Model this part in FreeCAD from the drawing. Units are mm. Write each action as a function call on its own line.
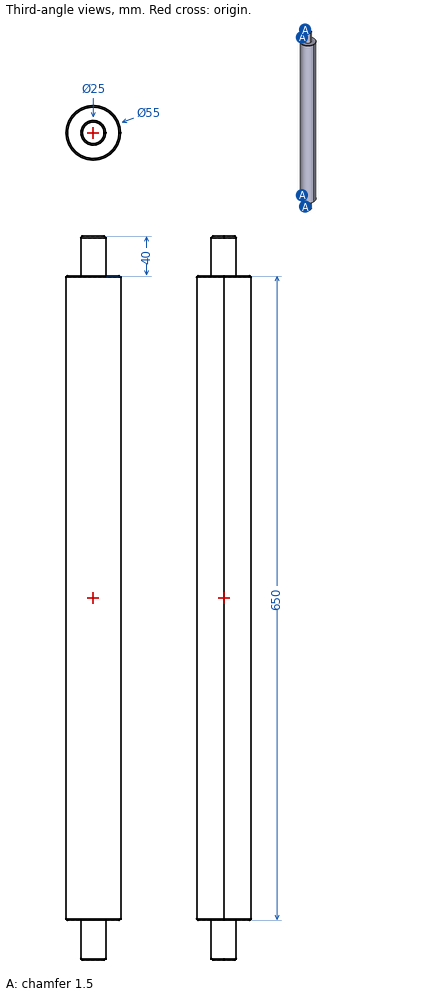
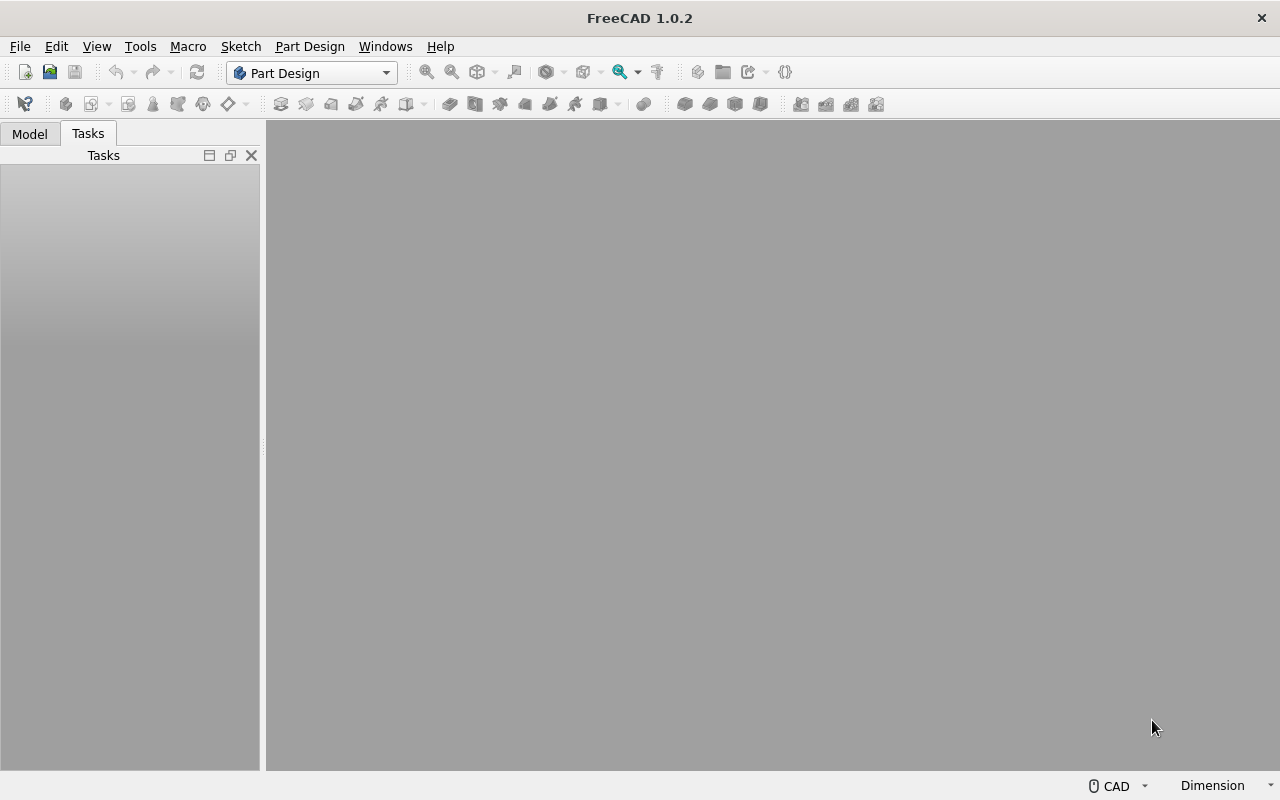
click(25, 72)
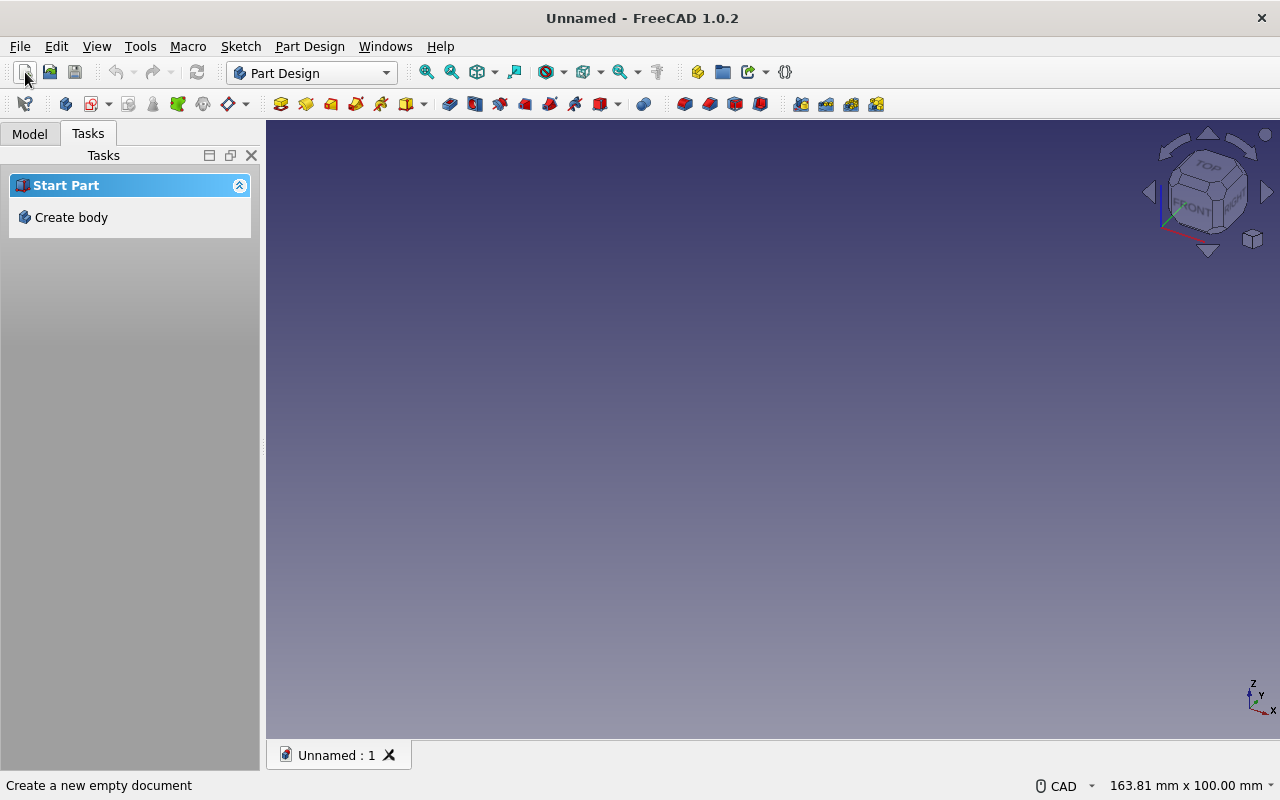
click(90, 104)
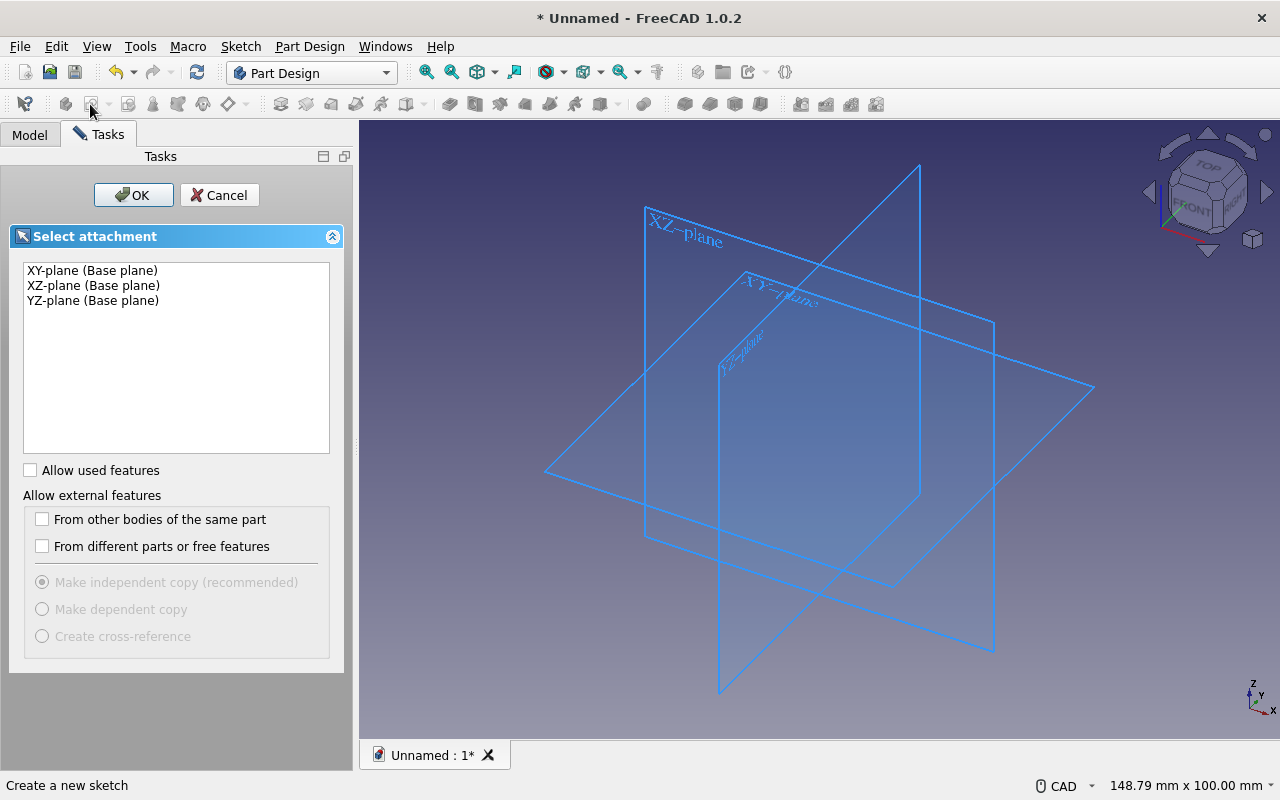
click(84, 270)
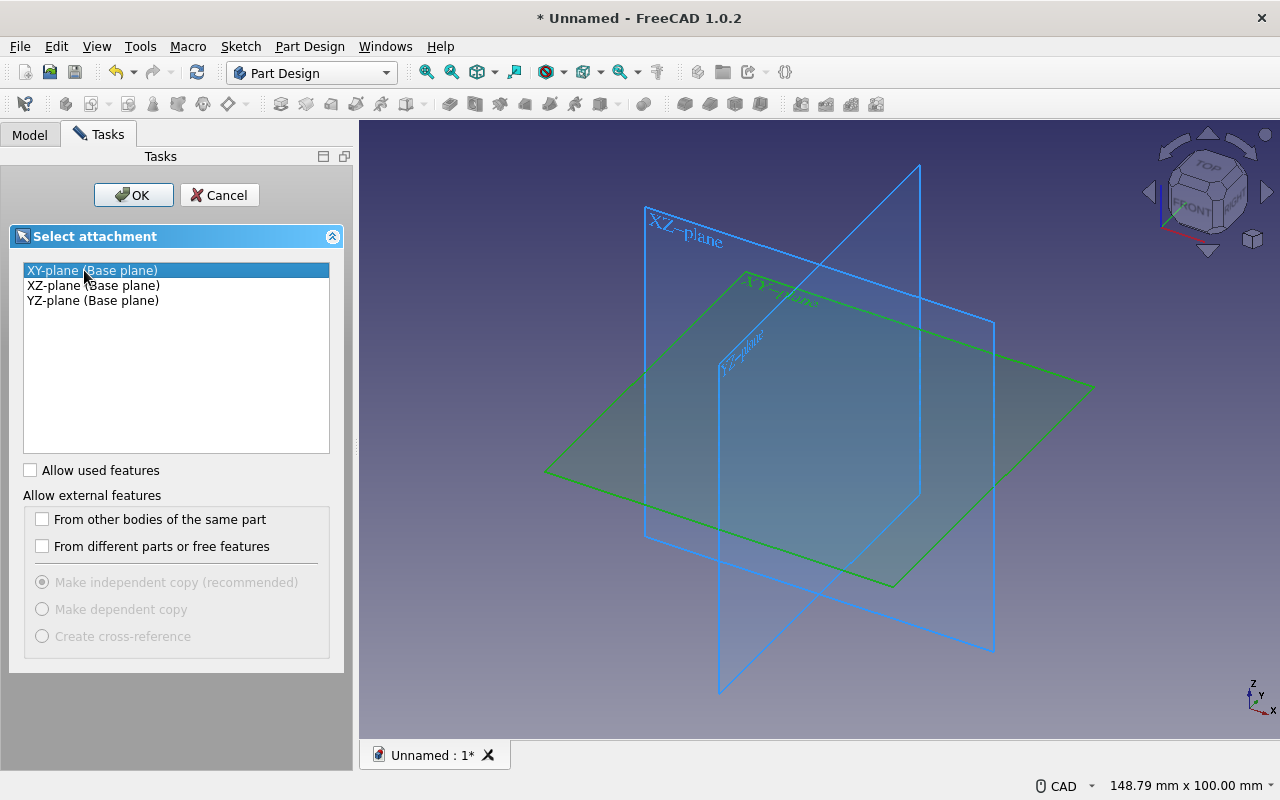
click(134, 195)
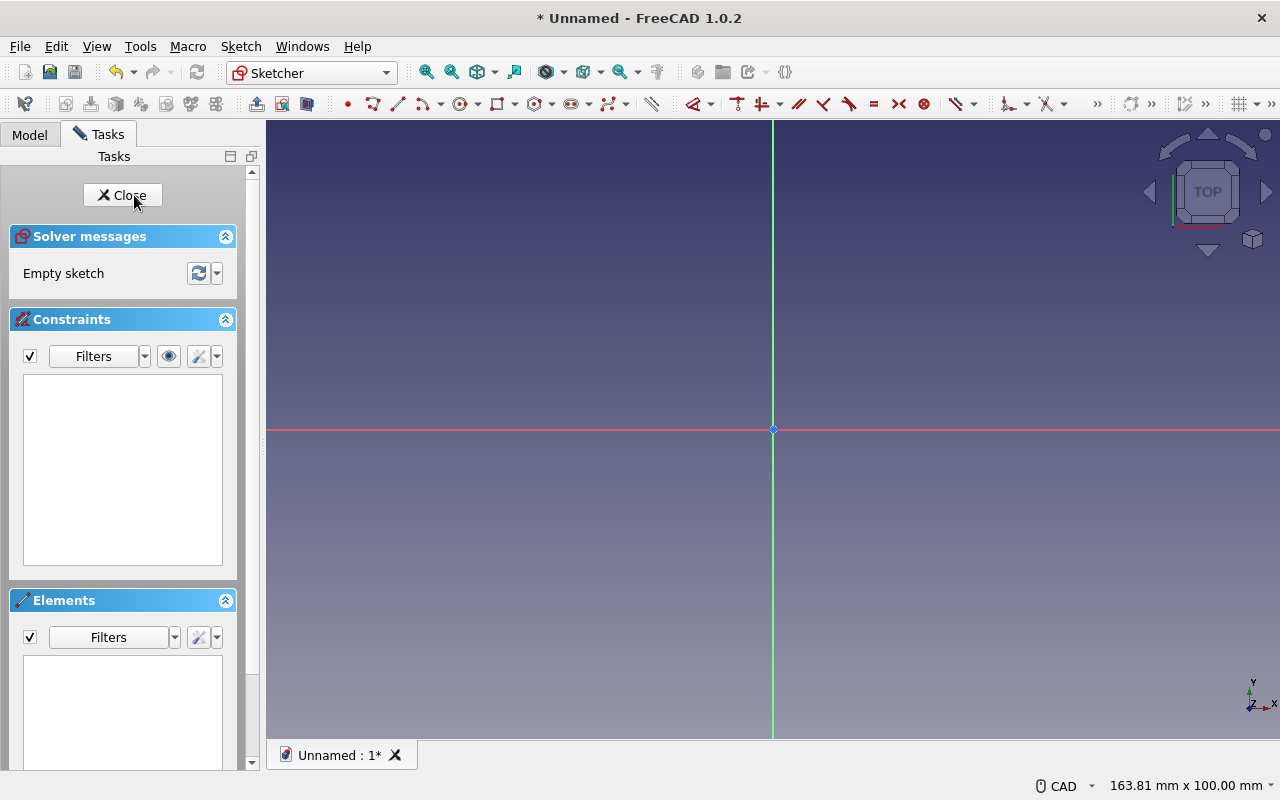
click(460, 104)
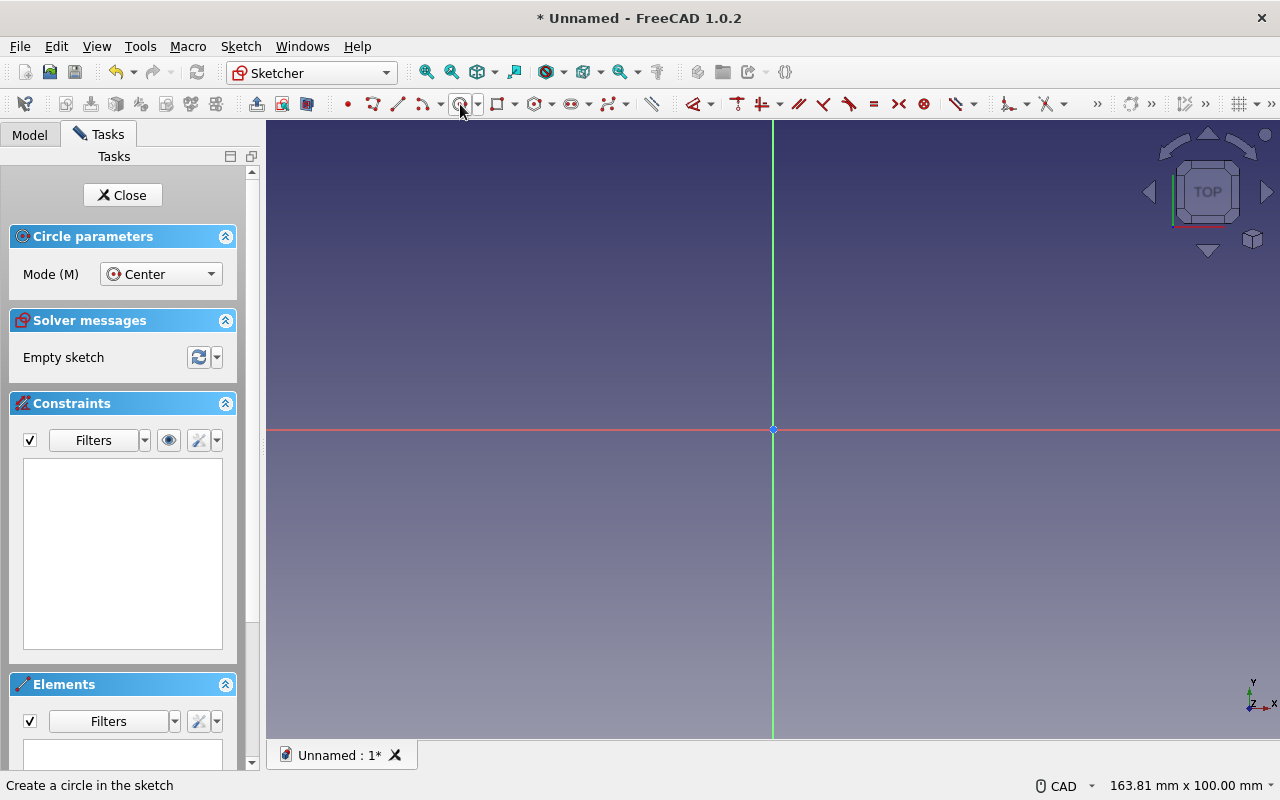
click(773, 430)
move(893, 309)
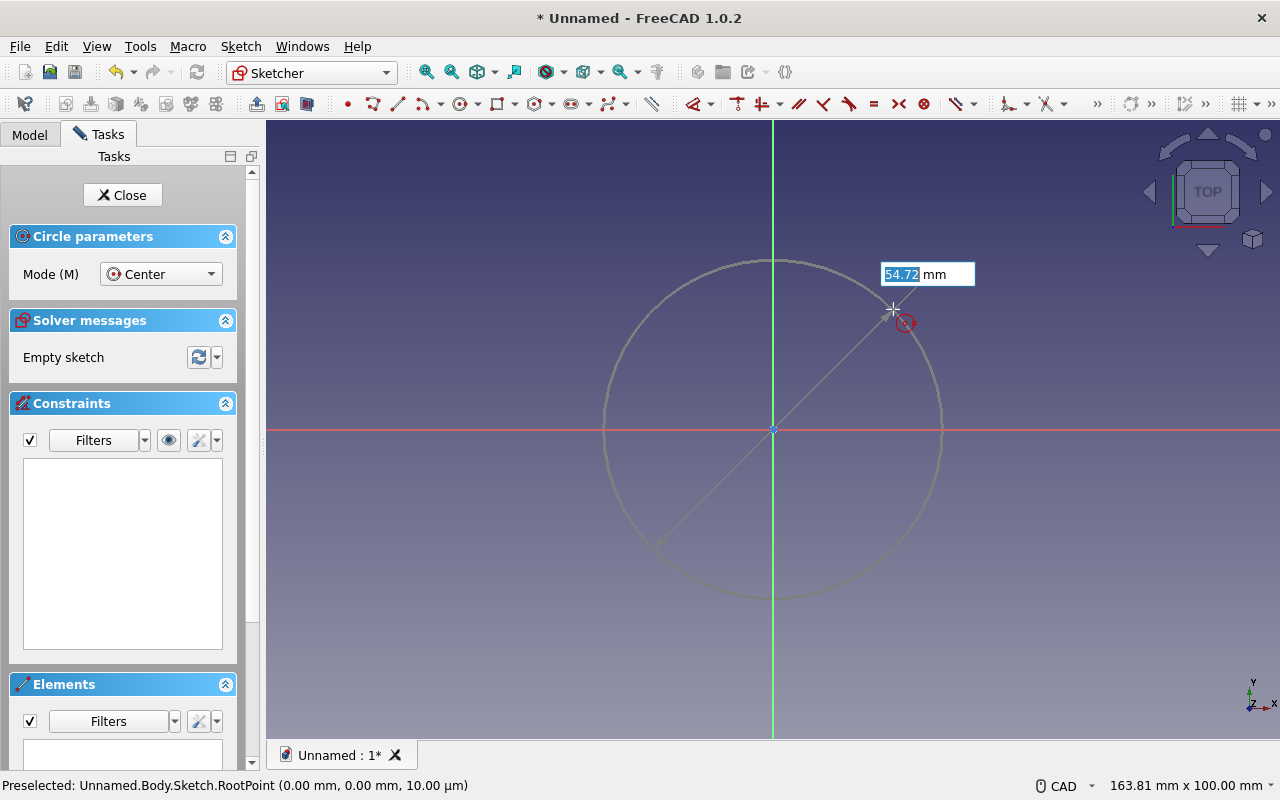
text(55)
key(Return)
key(Escape)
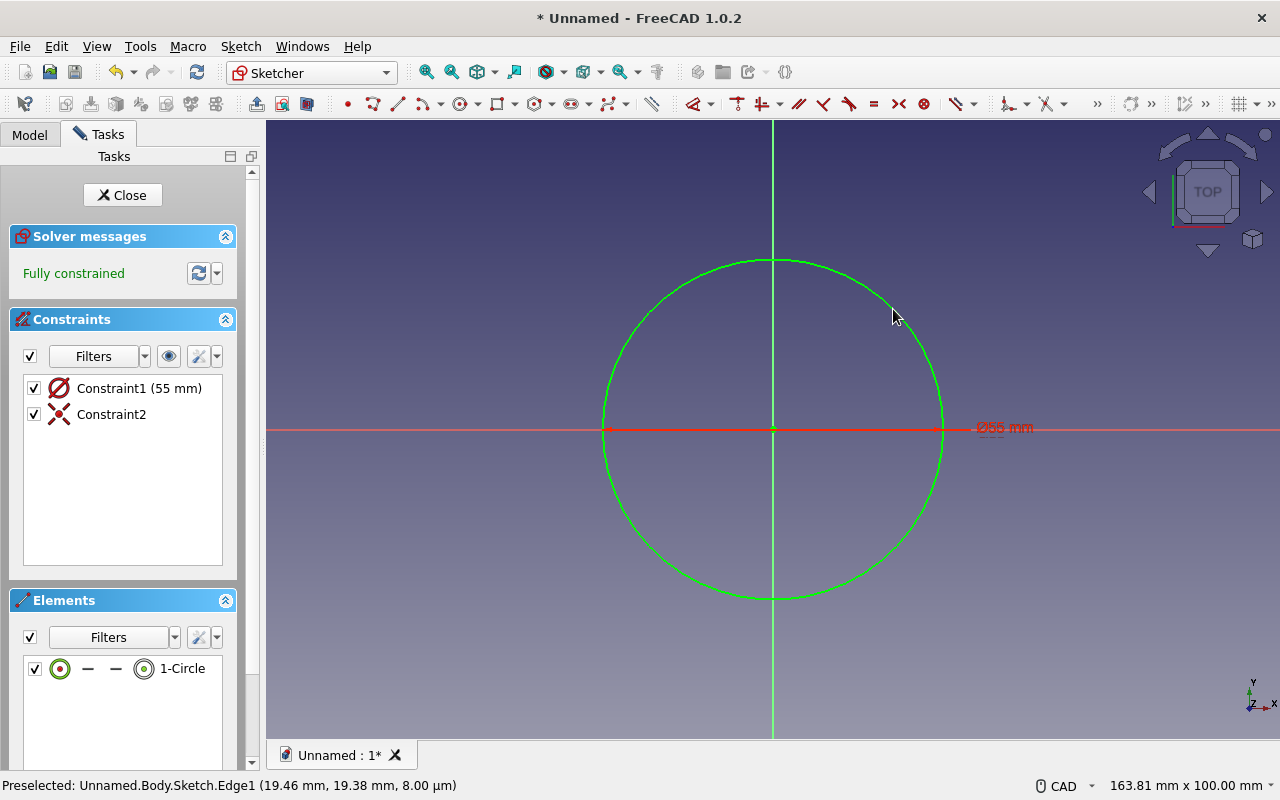
click(123, 195)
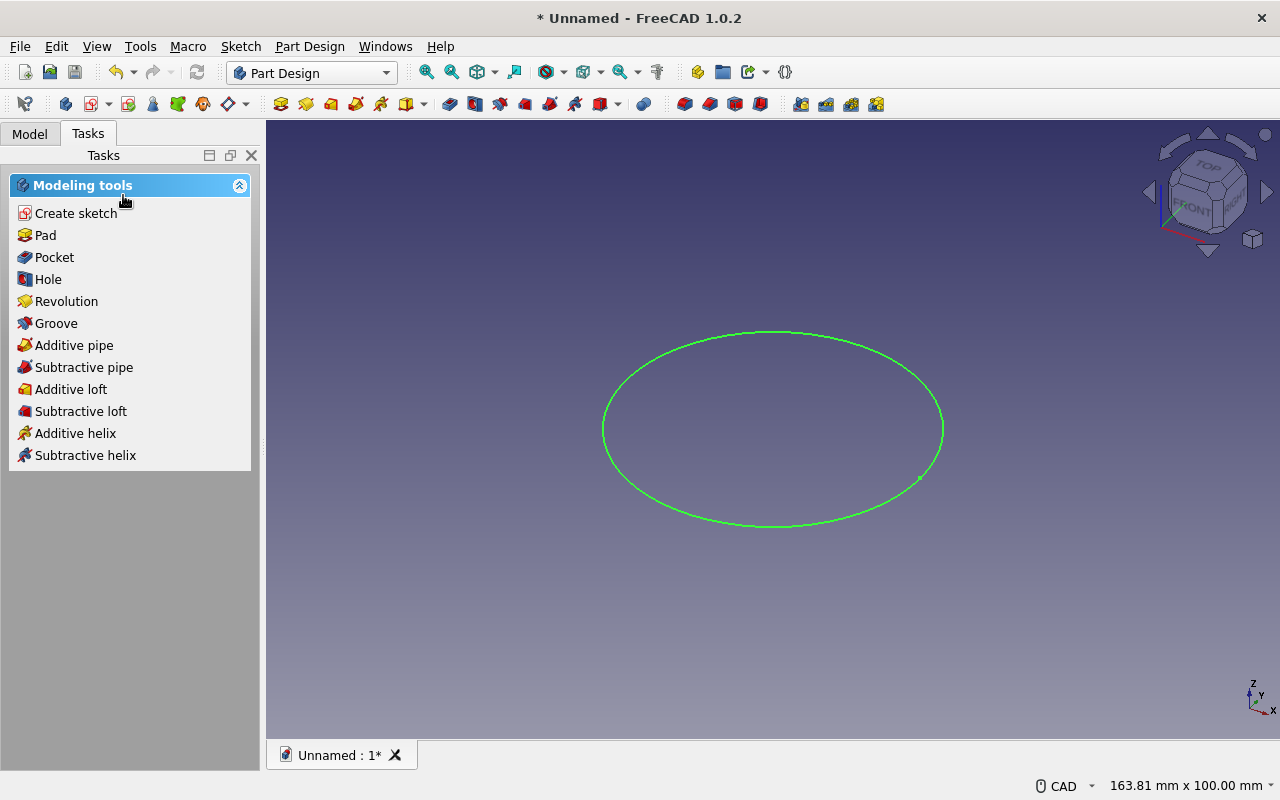
click(281, 104)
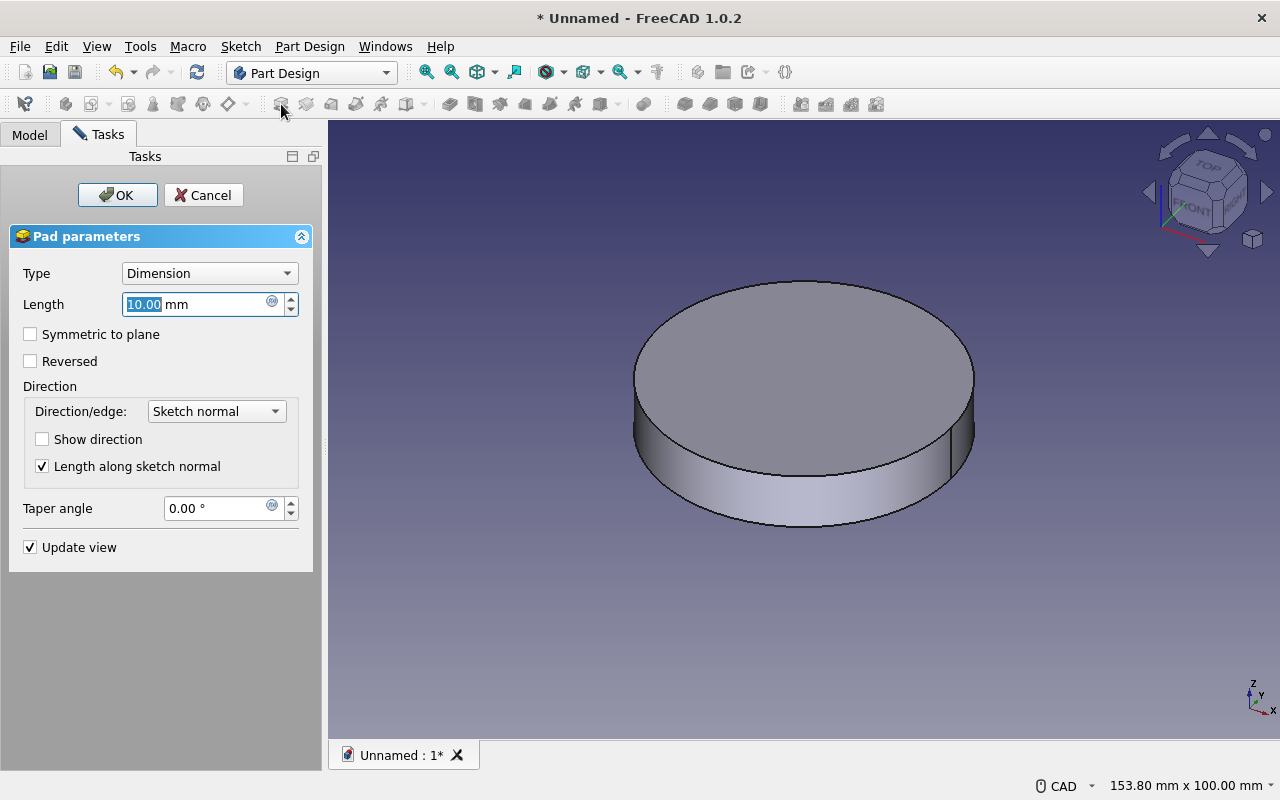
text(650)
key(Tab)